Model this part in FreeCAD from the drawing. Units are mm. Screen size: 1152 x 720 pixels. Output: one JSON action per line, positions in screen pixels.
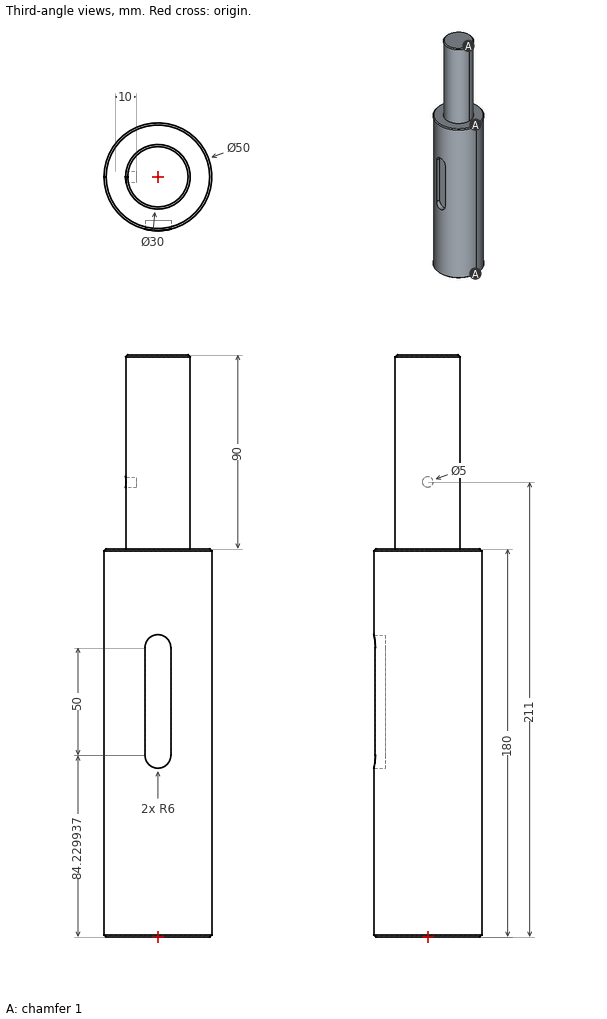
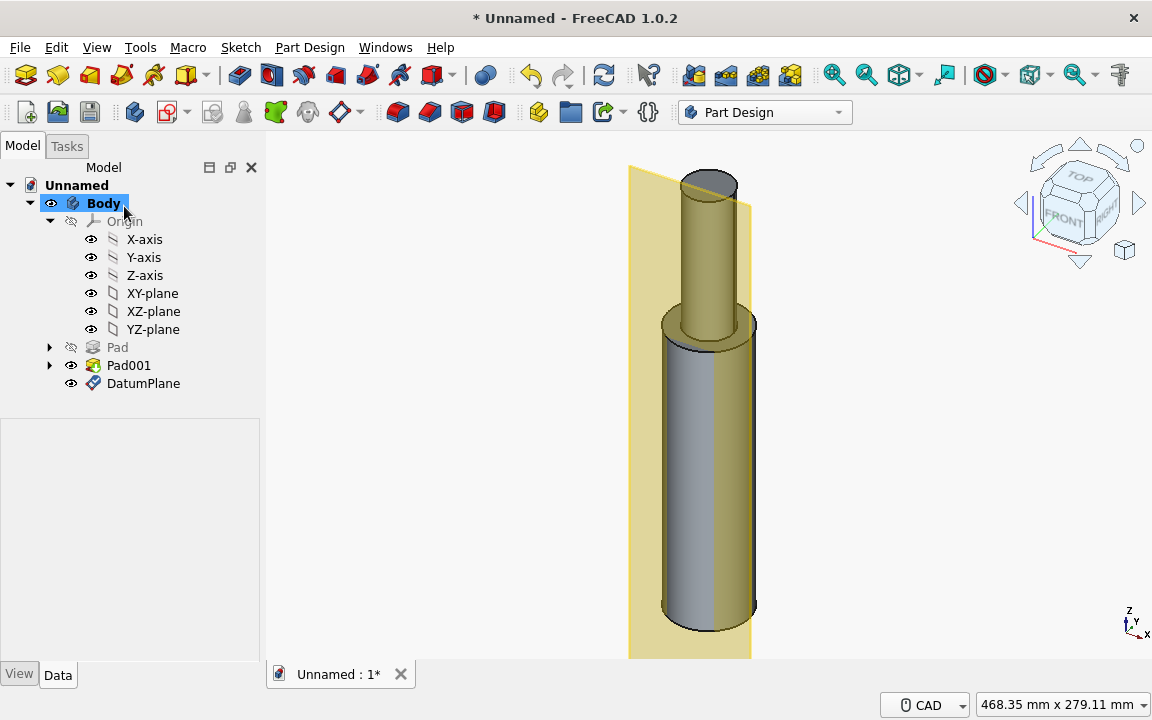
{"action": "left_click", "coordinate": [116, 383]}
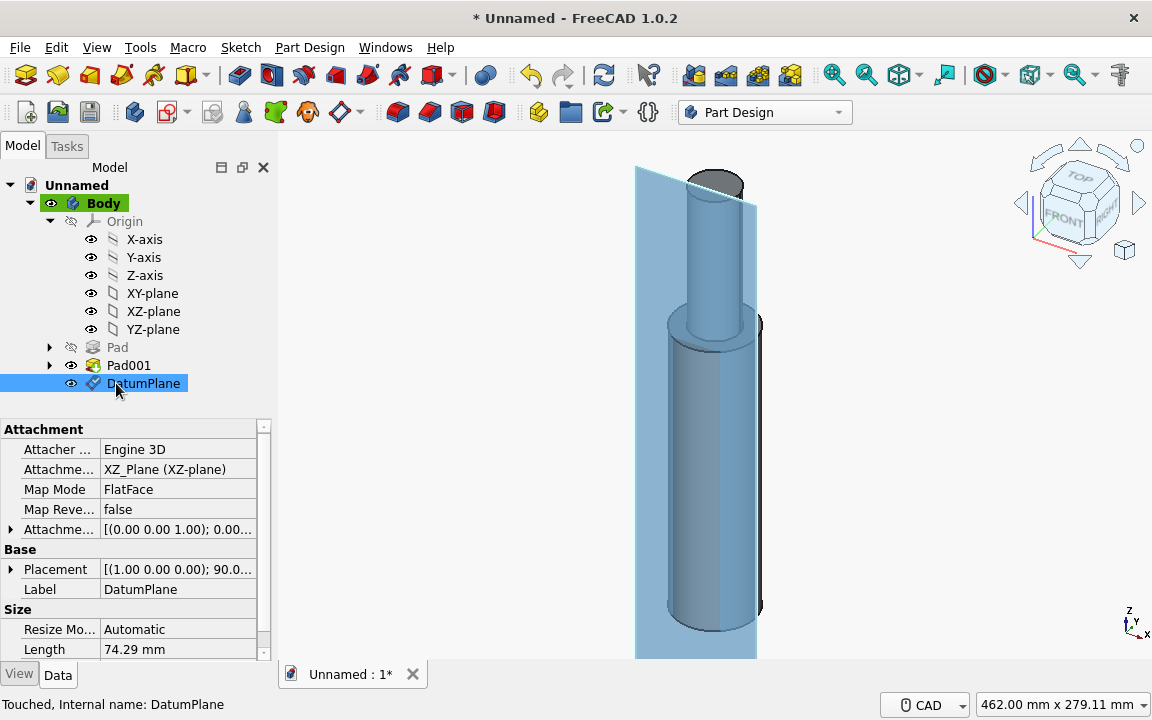
{"action": "left_click", "coordinate": [168, 112]}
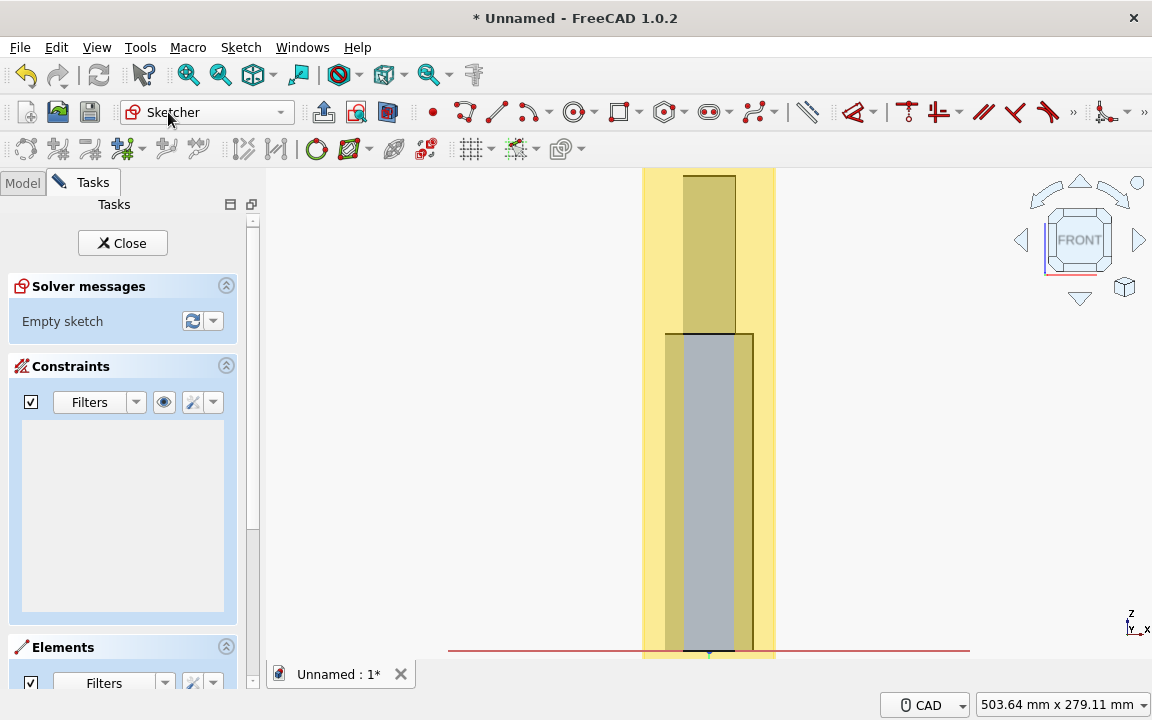
{"action": "key", "text": "q s"}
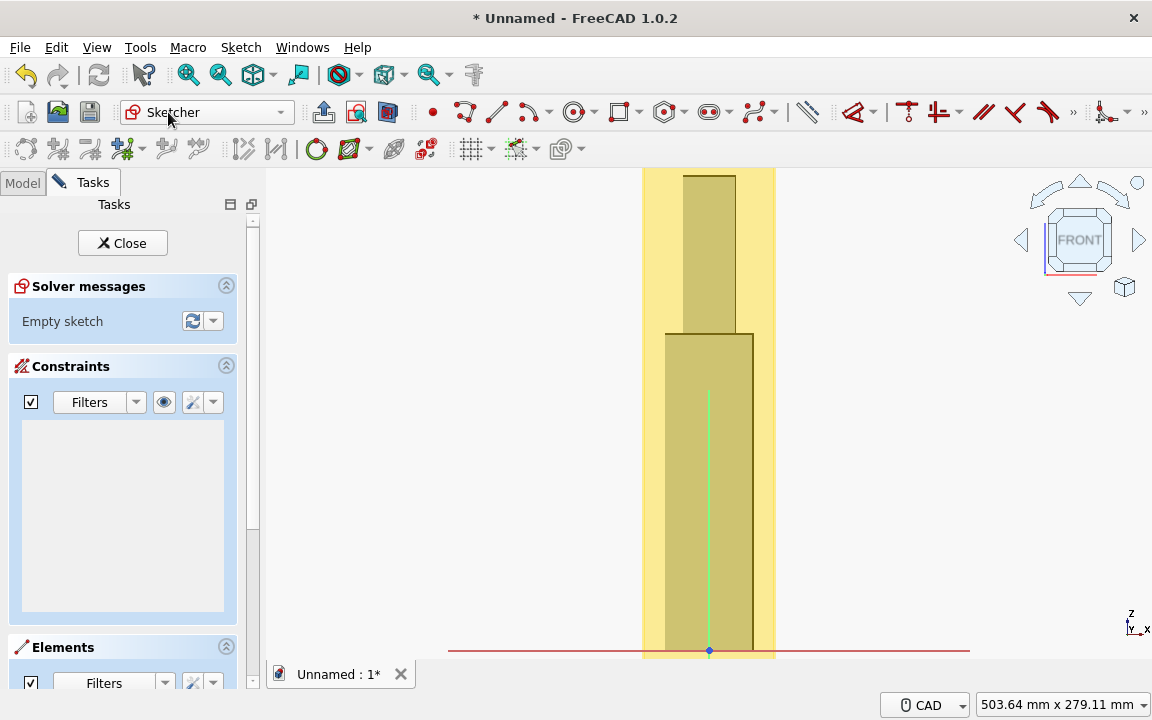
{"action": "scroll", "coordinate": [331, 196], "scroll_direction": "down", "scroll_amount": 1}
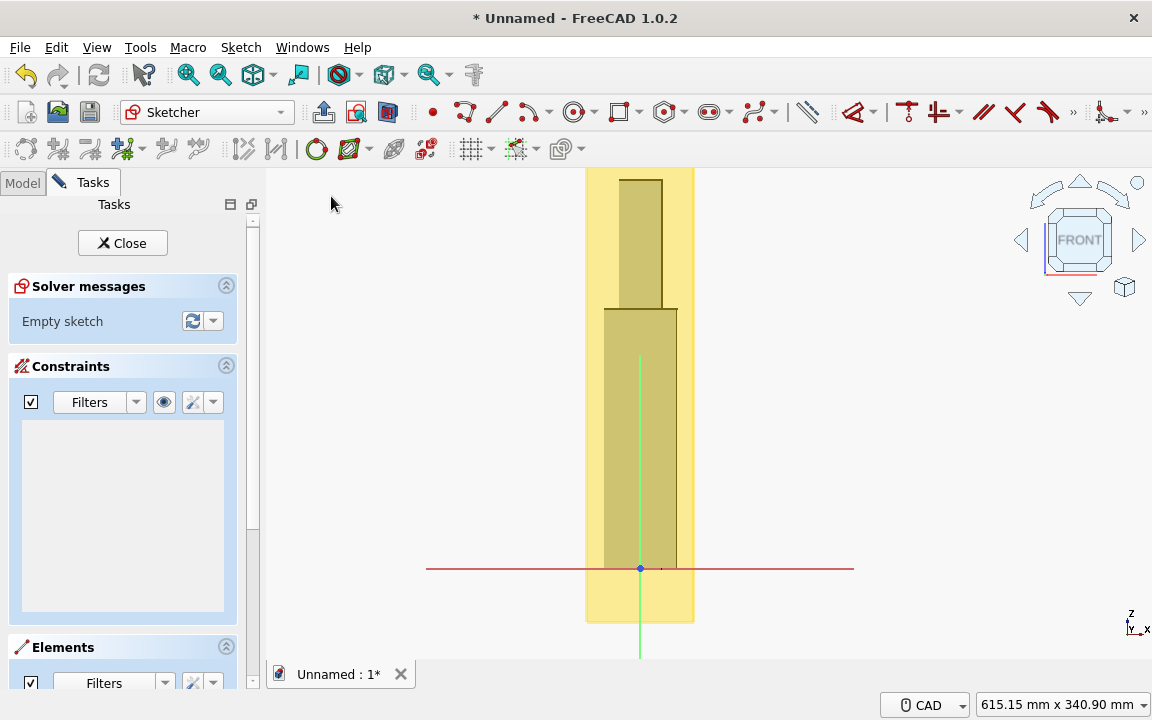
{"action": "scroll", "coordinate": [640, 577], "scroll_direction": "up", "scroll_amount": 2}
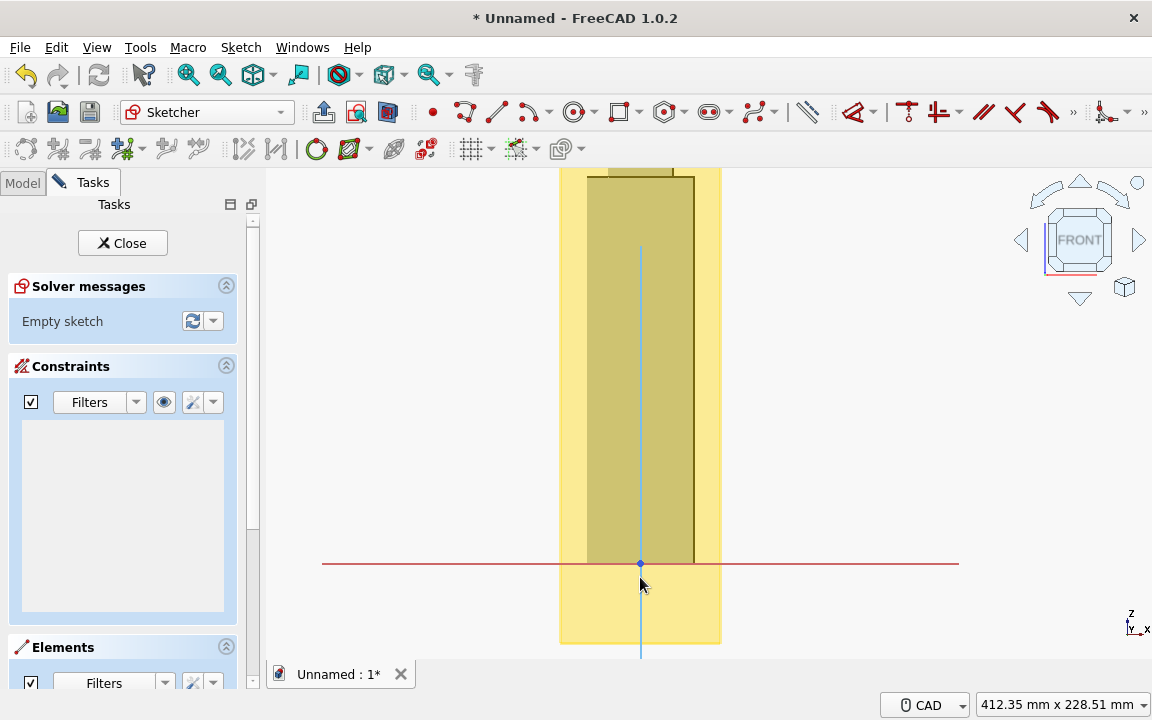
{"action": "key", "text": "g s"}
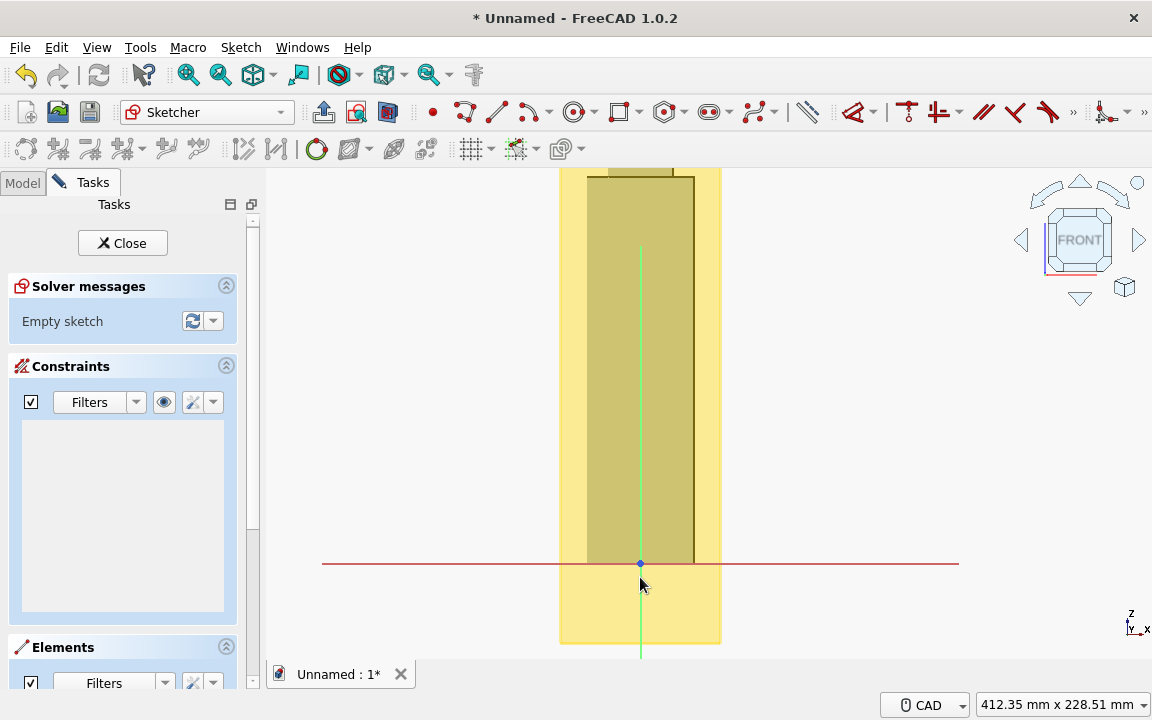
{"action": "scroll", "coordinate": [641, 383], "scroll_direction": "up", "scroll_amount": 3}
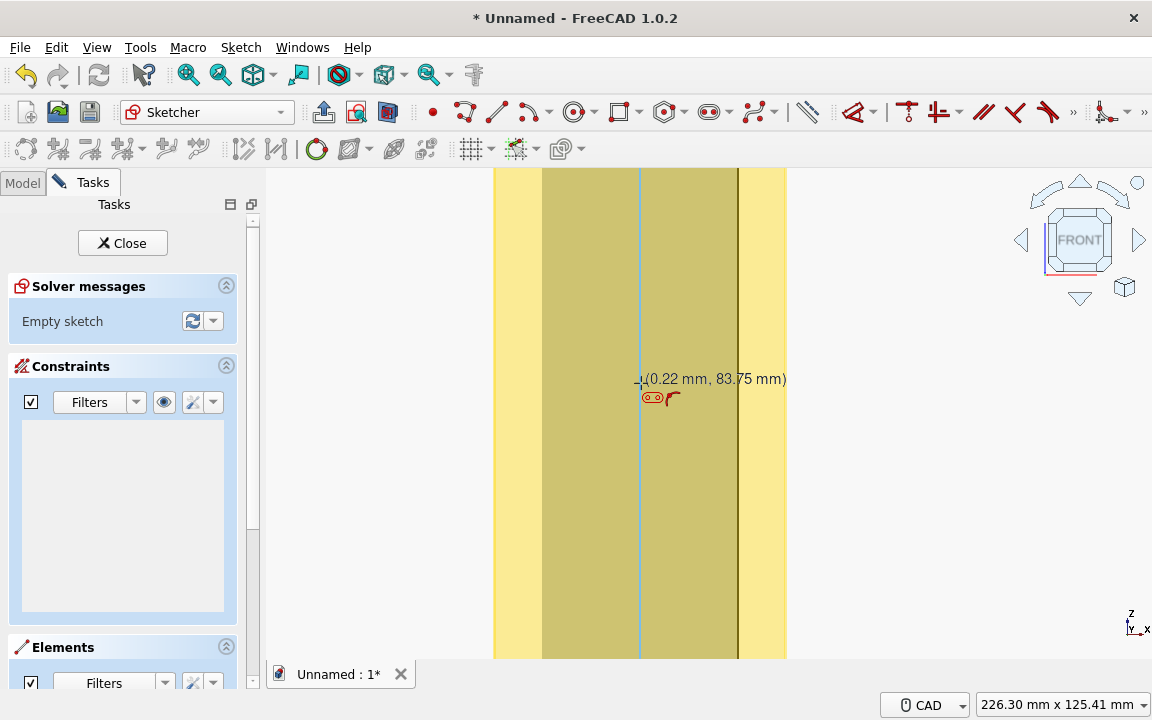
{"action": "left_click", "coordinate": [640, 383]}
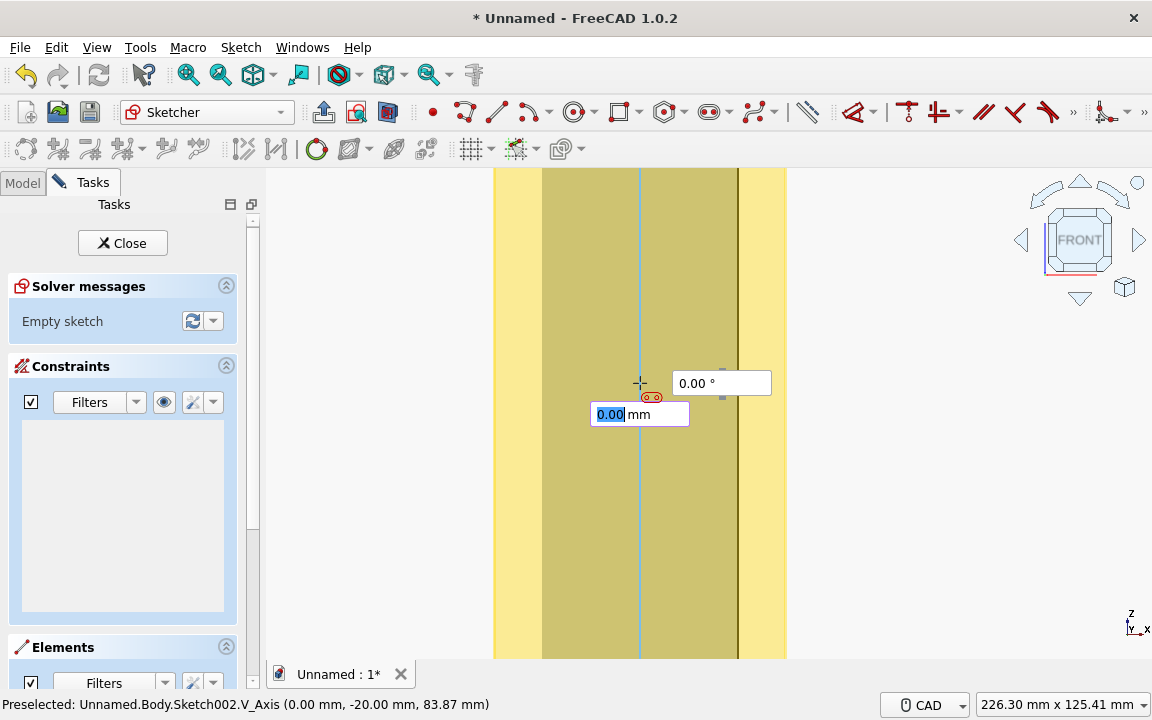
{"action": "scroll", "coordinate": [641, 384], "scroll_direction": "down", "scroll_amount": 3}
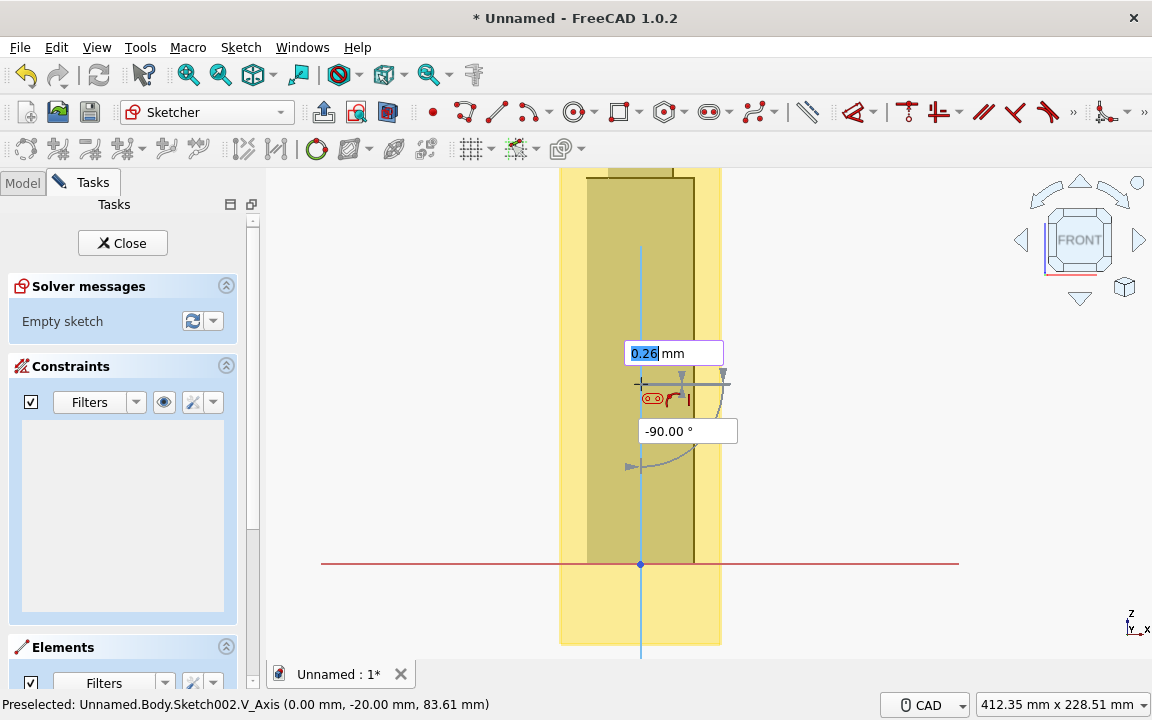
{"action": "left_click", "coordinate": [650, 276]}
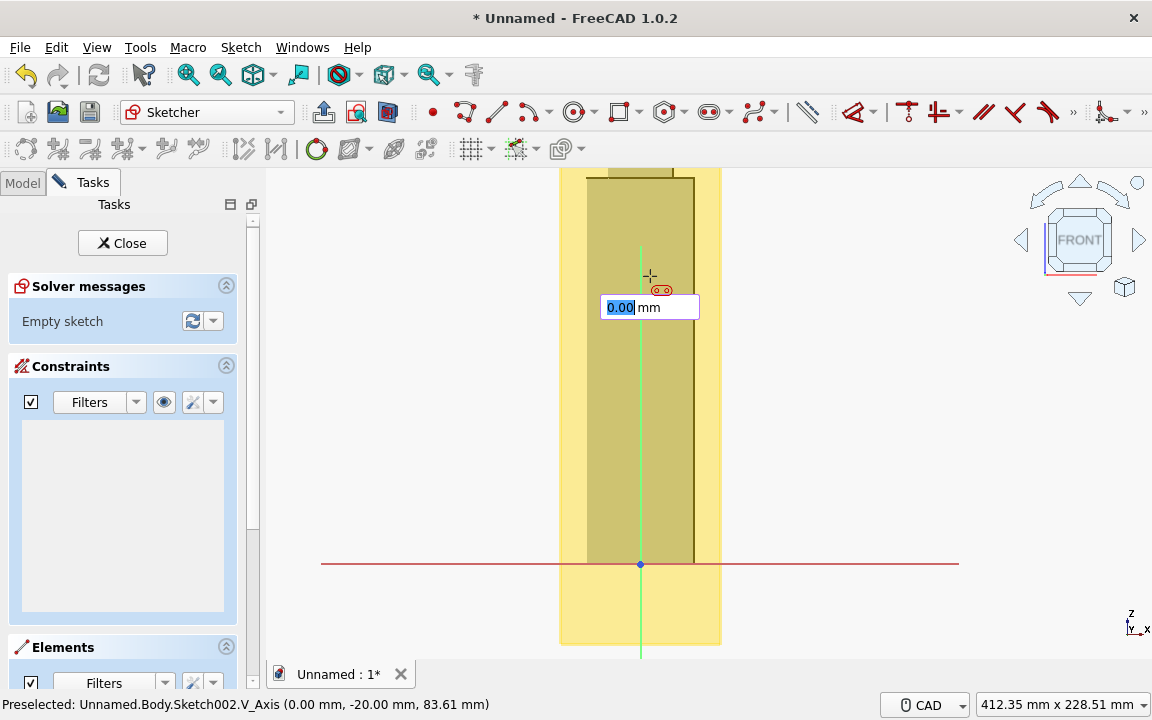
{"action": "scroll", "coordinate": [653, 330], "scroll_direction": "up", "scroll_amount": 2}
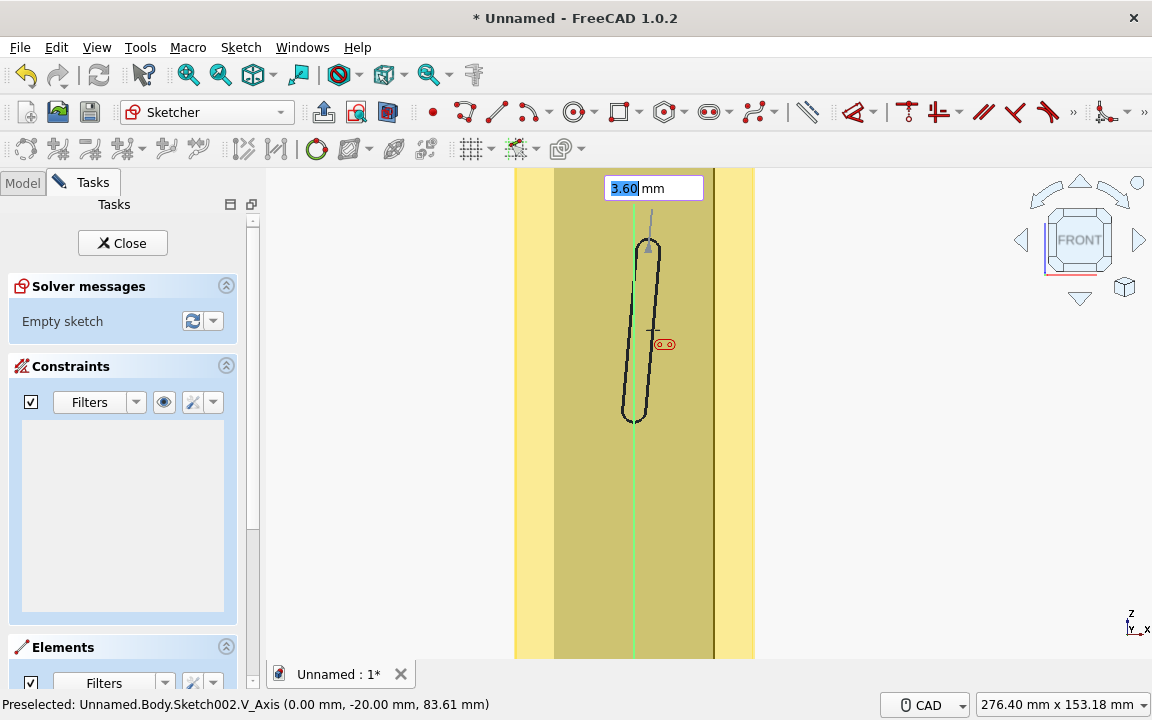
{"action": "left_click", "coordinate": [653, 329]}
{"action": "key", "text": "Escape"}